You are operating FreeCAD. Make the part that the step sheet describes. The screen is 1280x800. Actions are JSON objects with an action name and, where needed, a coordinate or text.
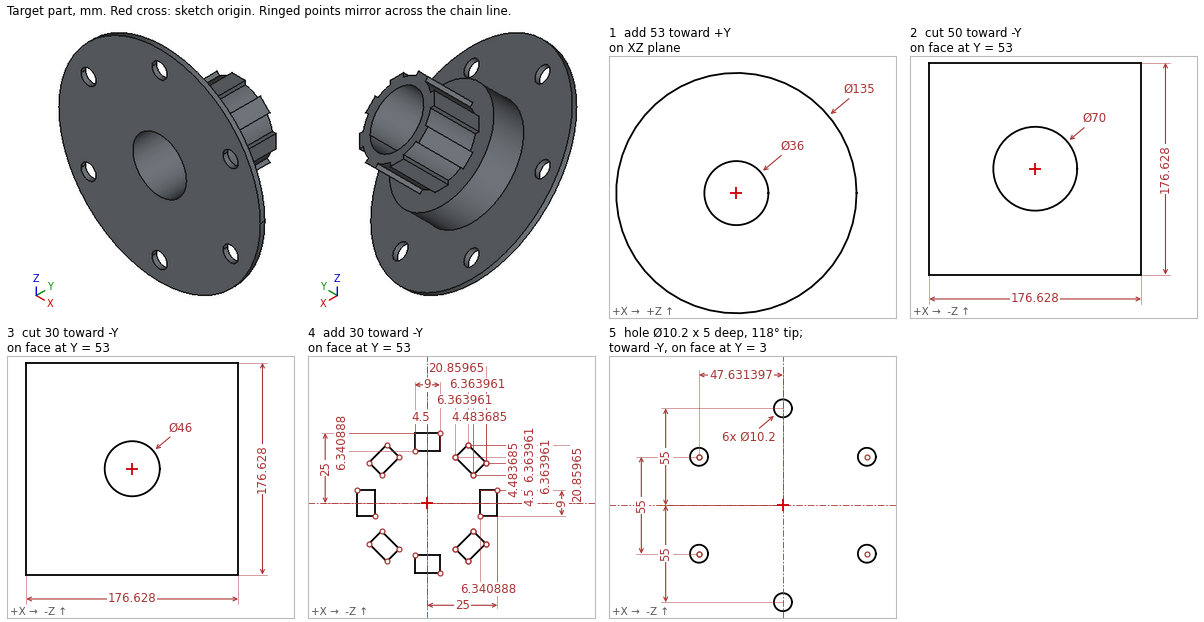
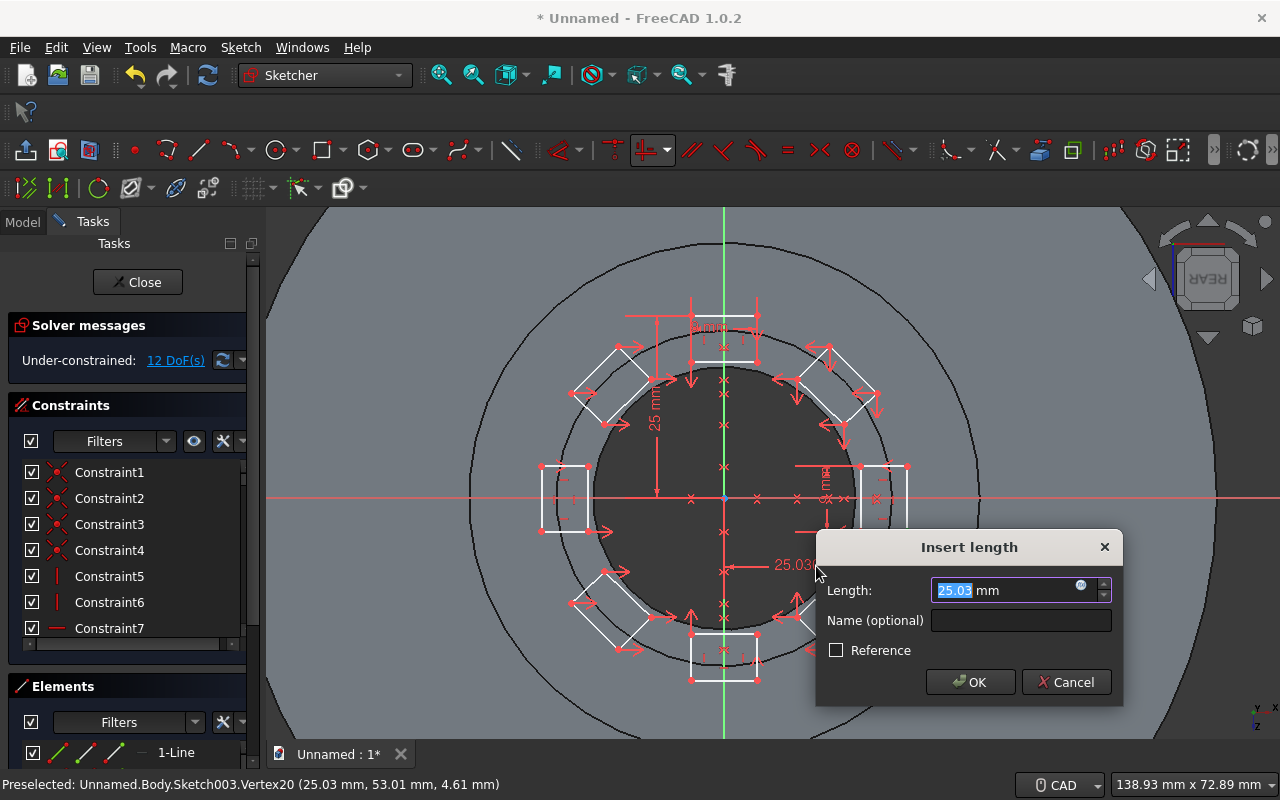
{"action": "type", "text": "25"}
{"action": "key", "text": "Return"}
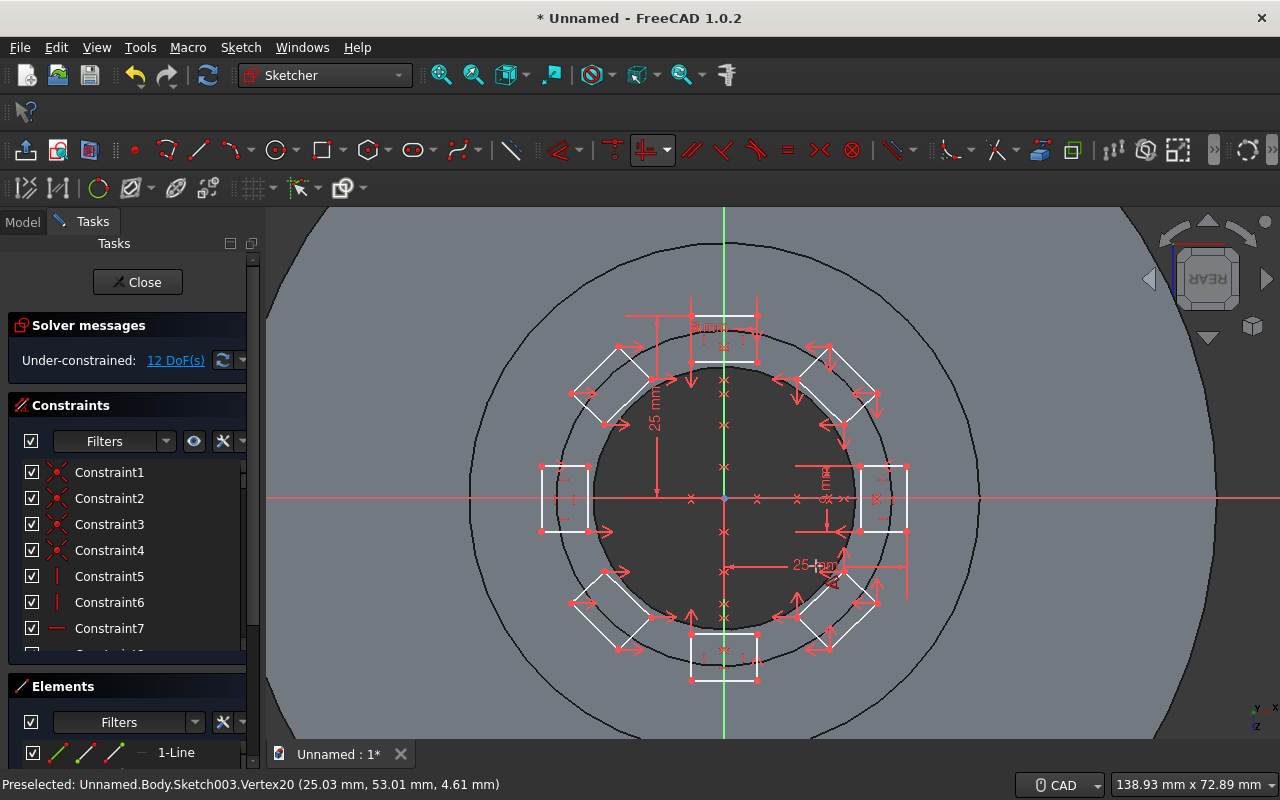
{"action": "left_click", "coordinate": [691, 316]}
{"action": "left_click", "coordinate": [708, 282]}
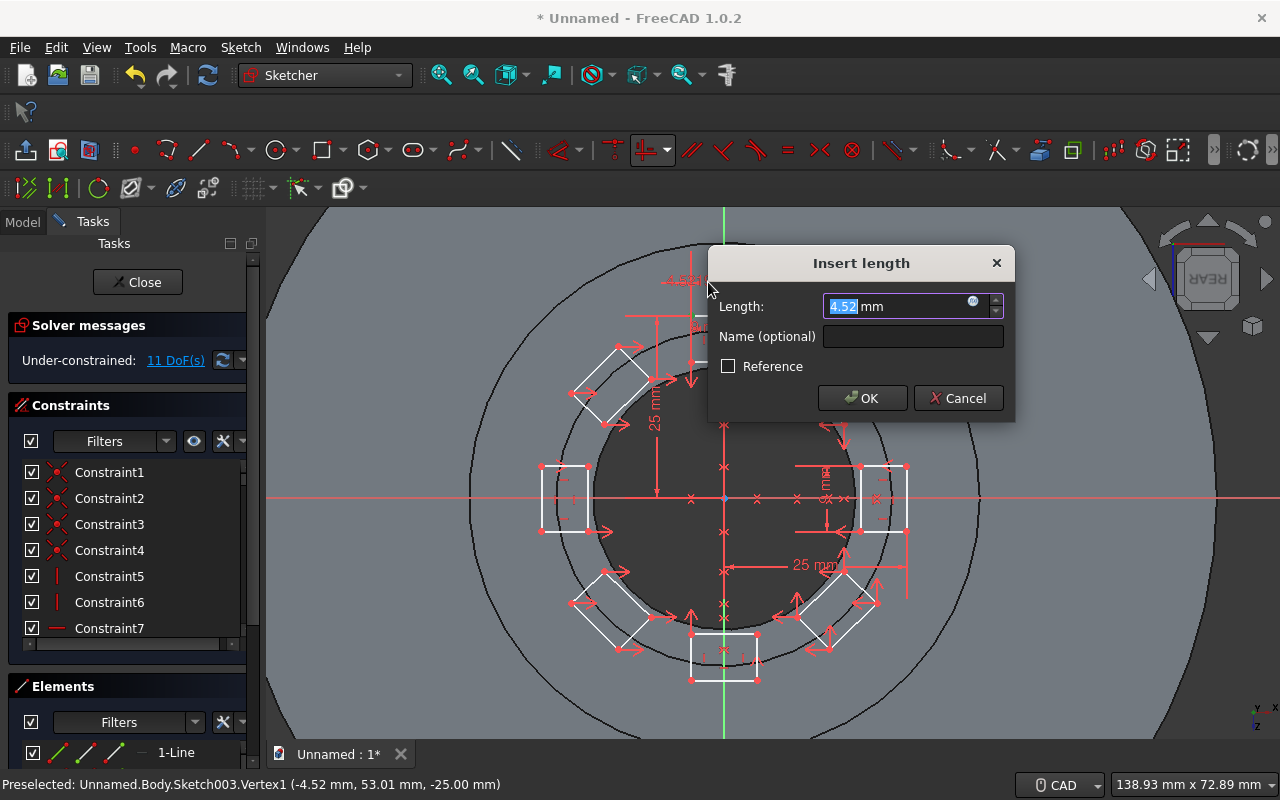
{"action": "type", "text": "4.5"}
{"action": "key", "text": "Return"}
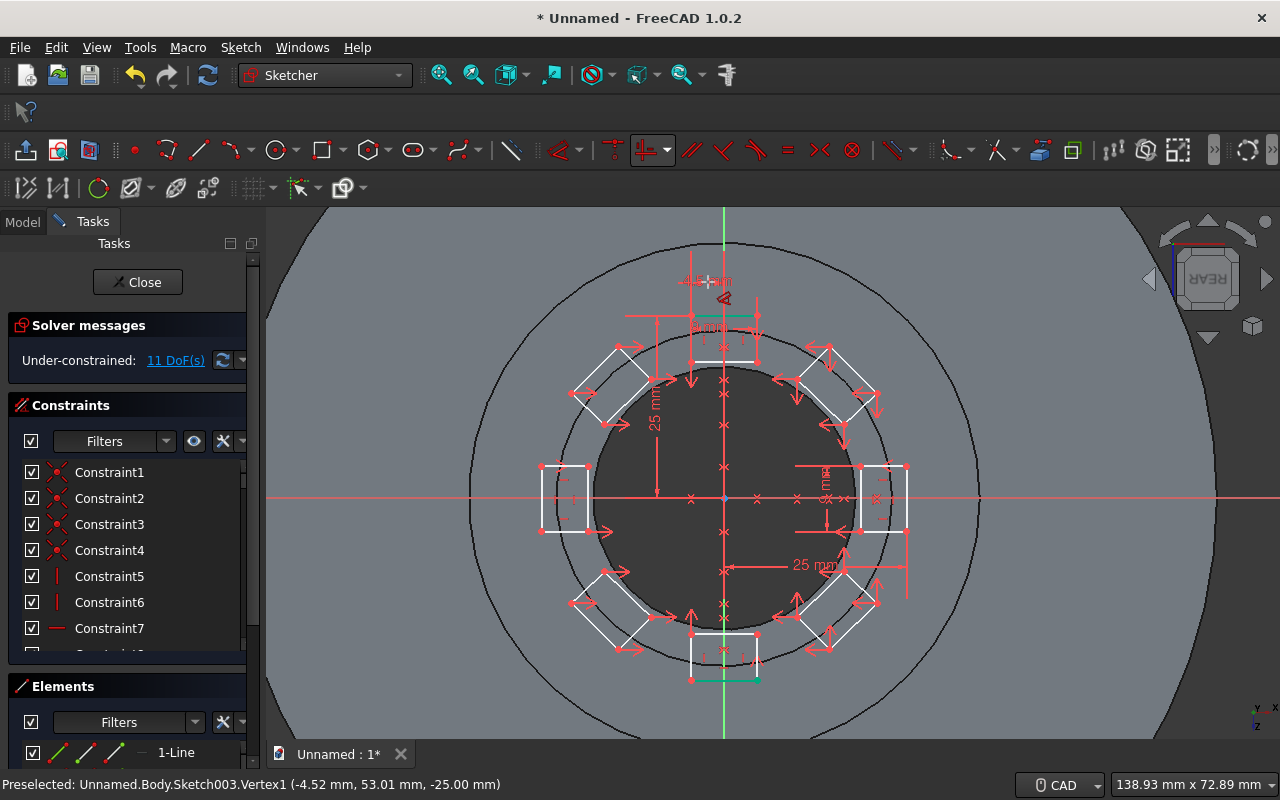
{"action": "left_click", "coordinate": [861, 466]}
{"action": "left_click", "coordinate": [690, 482]}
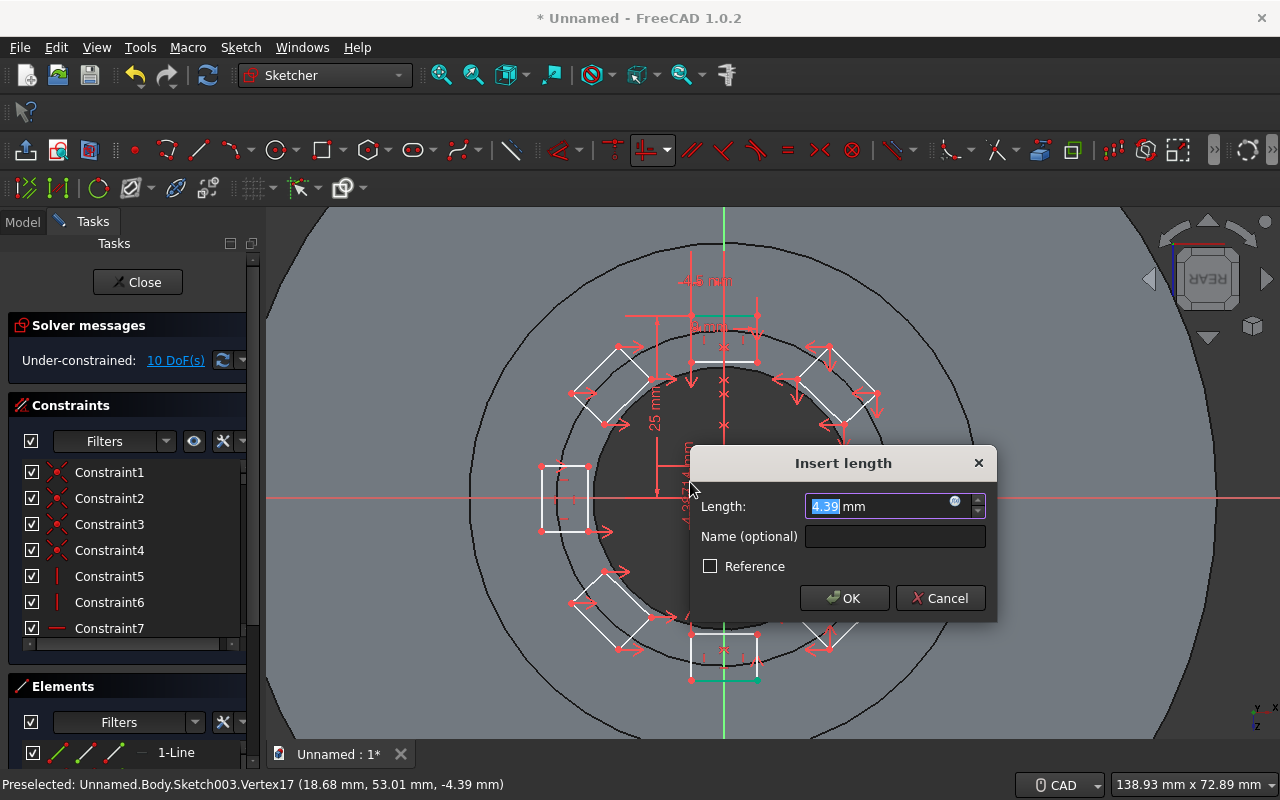
{"action": "type", "text": "4.5"}
{"action": "key", "text": "Return"}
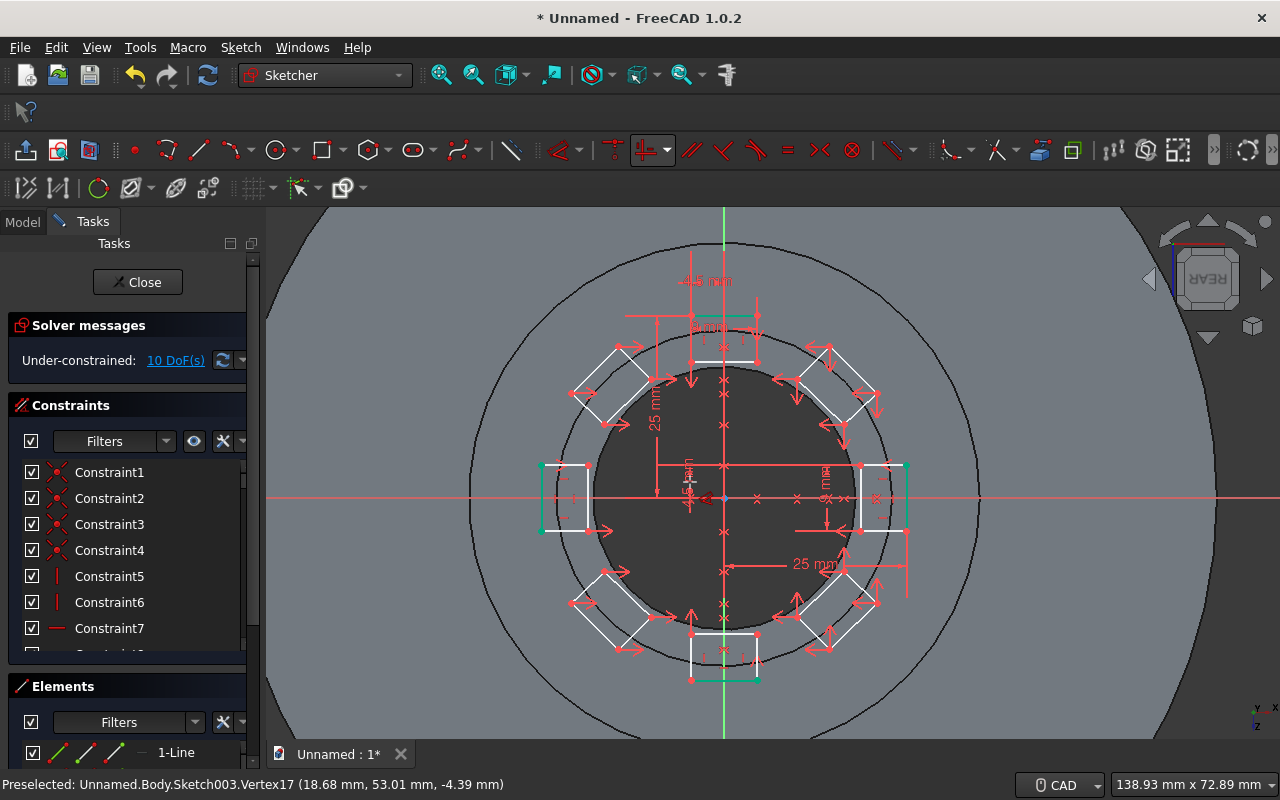
{"action": "left_click", "coordinate": [691, 330]}
{"action": "left_click", "coordinate": [657, 350]}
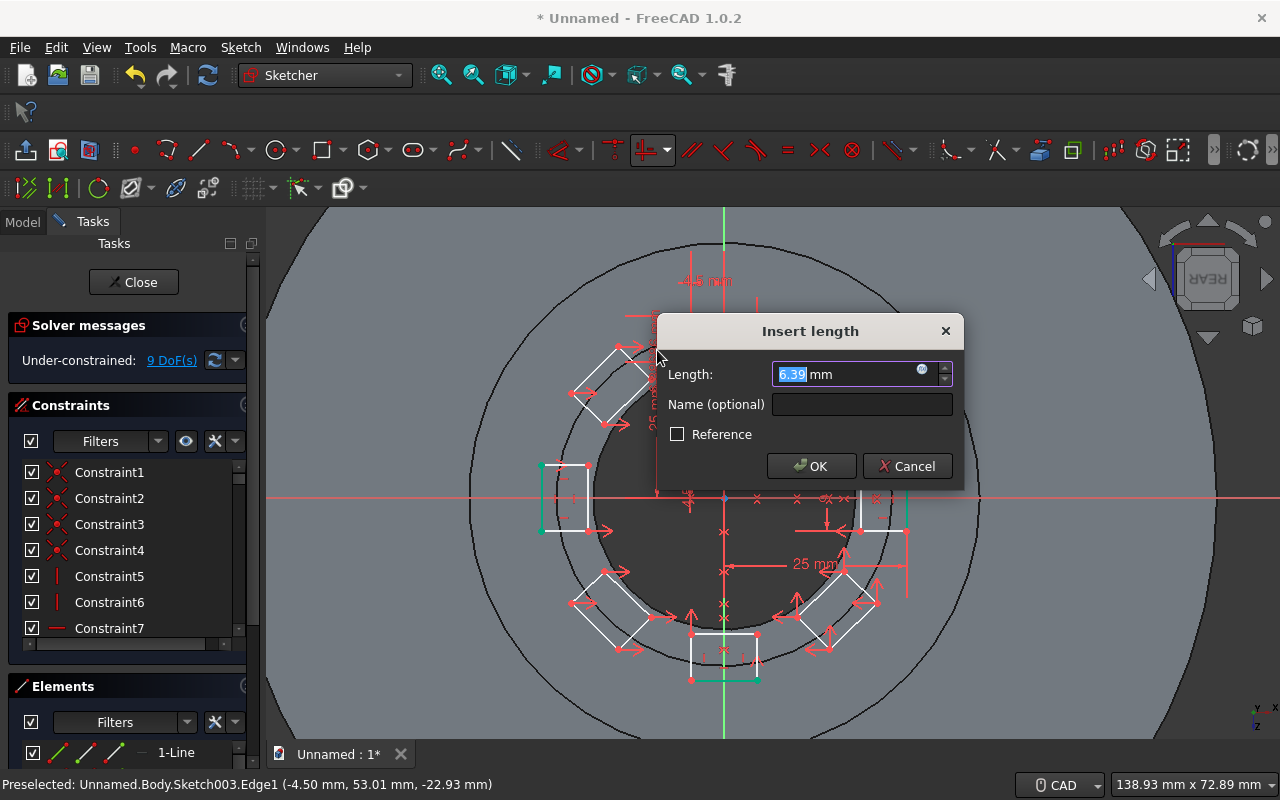
{"action": "type", "text": "6.340888"}
{"action": "key", "text": "Return"}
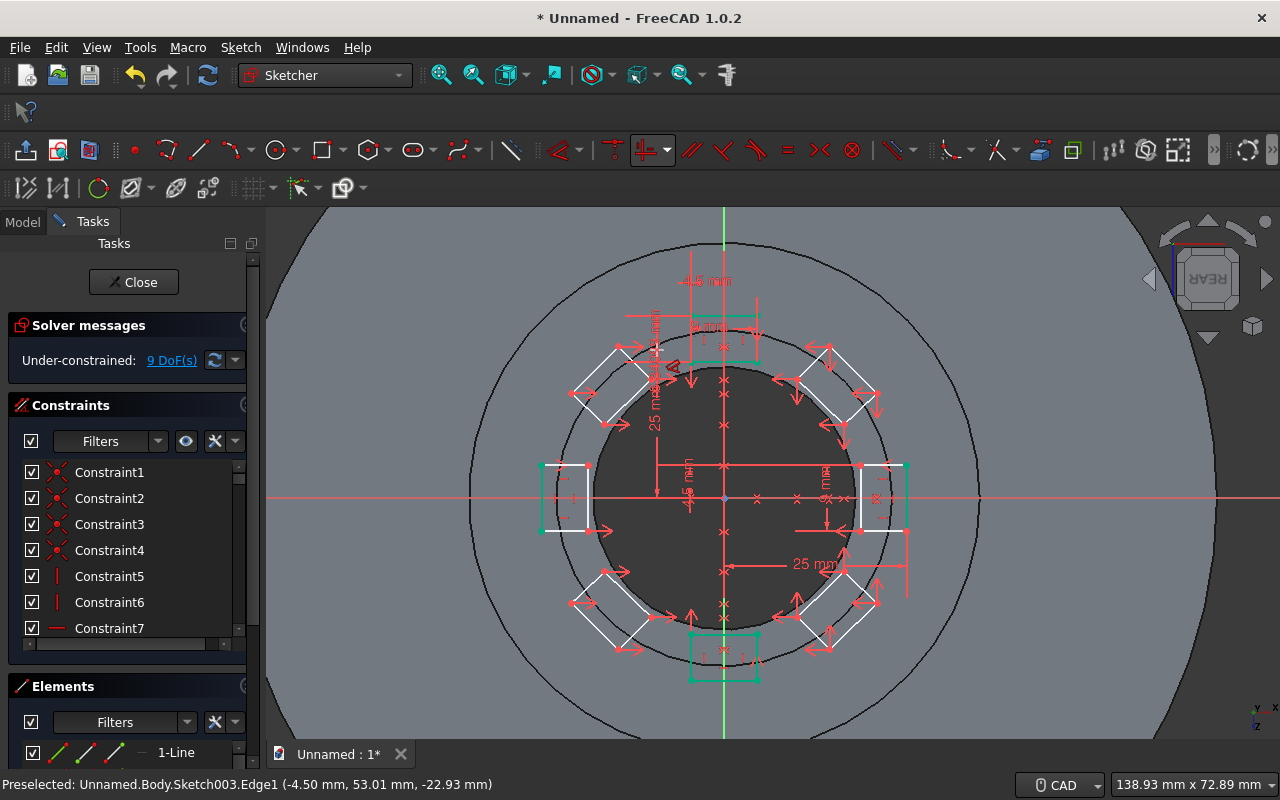
{"action": "left_click", "coordinate": [874, 531]}
{"action": "left_click", "coordinate": [894, 565]}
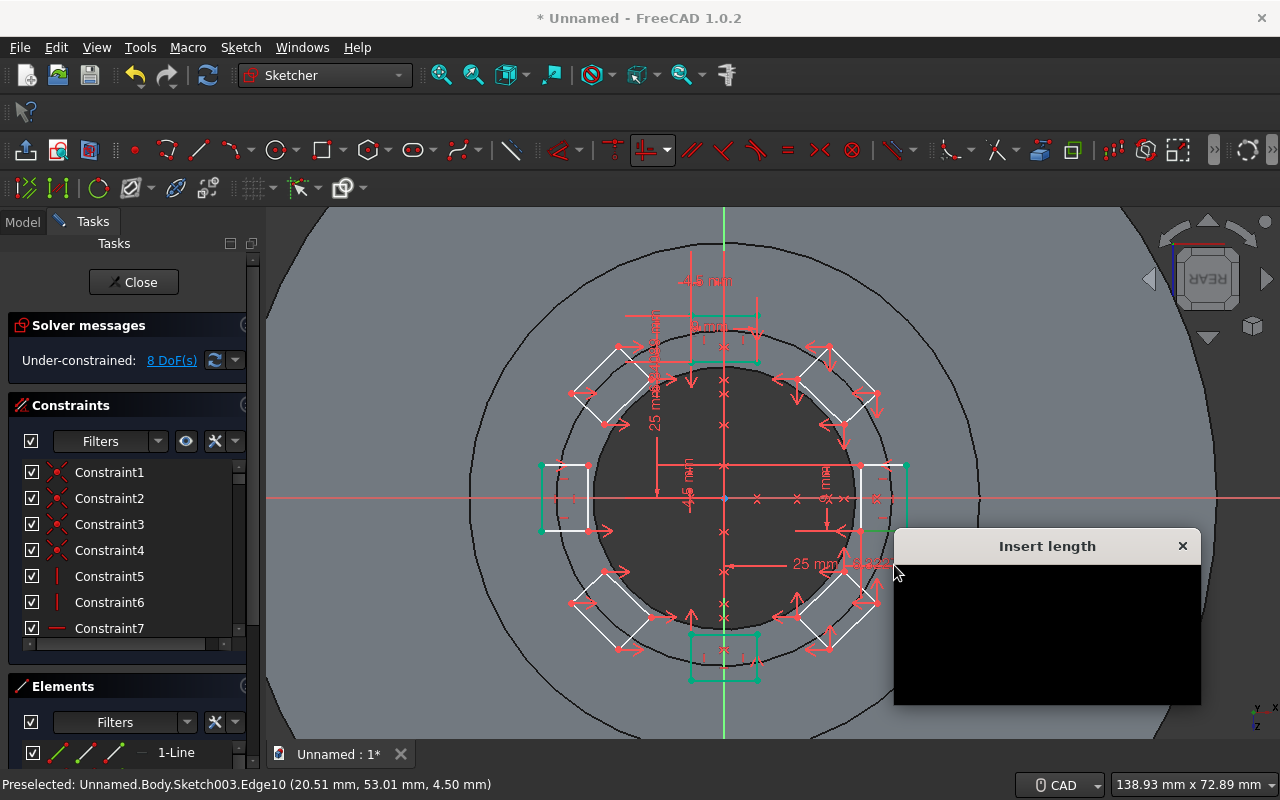
{"action": "type", "text": "6.340888"}
{"action": "key", "text": "Return"}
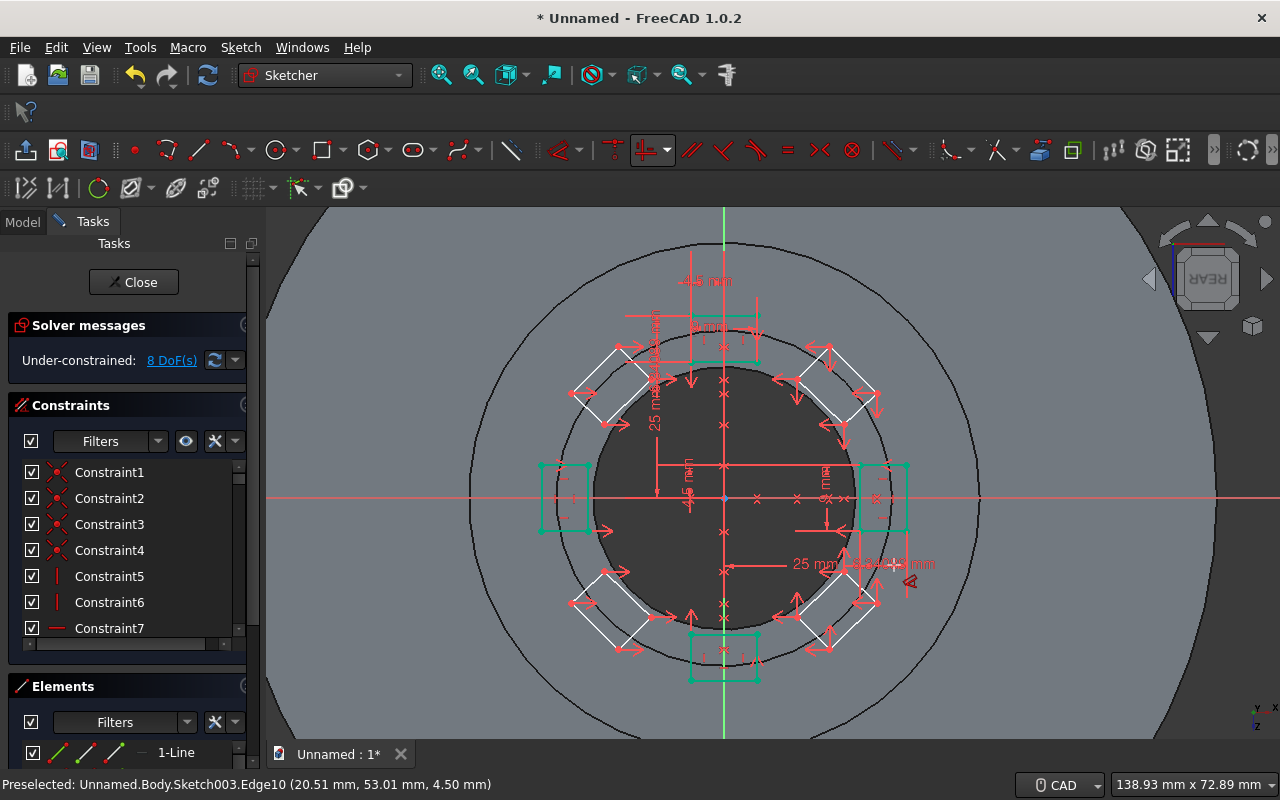
{"action": "left_click", "coordinate": [877, 393]}
{"action": "left_click", "coordinate": [801, 532]}